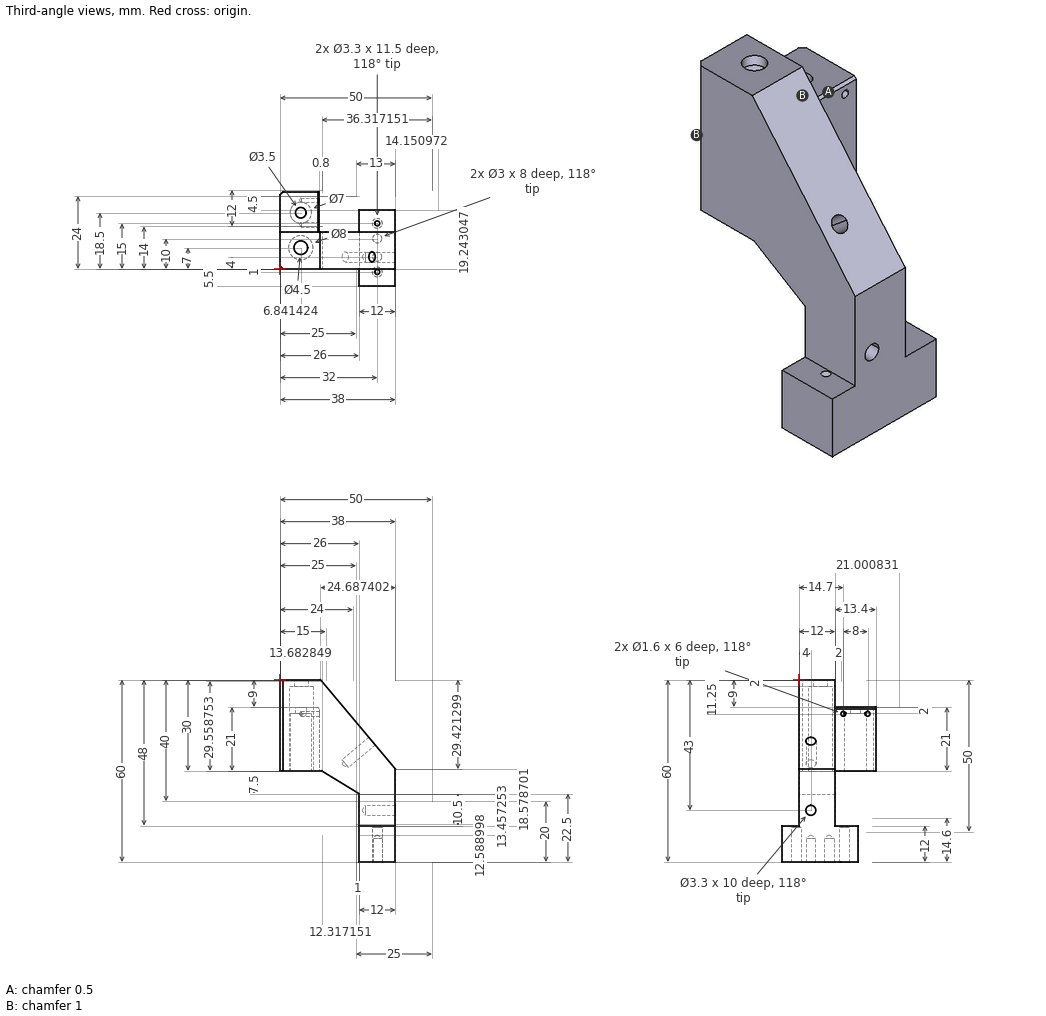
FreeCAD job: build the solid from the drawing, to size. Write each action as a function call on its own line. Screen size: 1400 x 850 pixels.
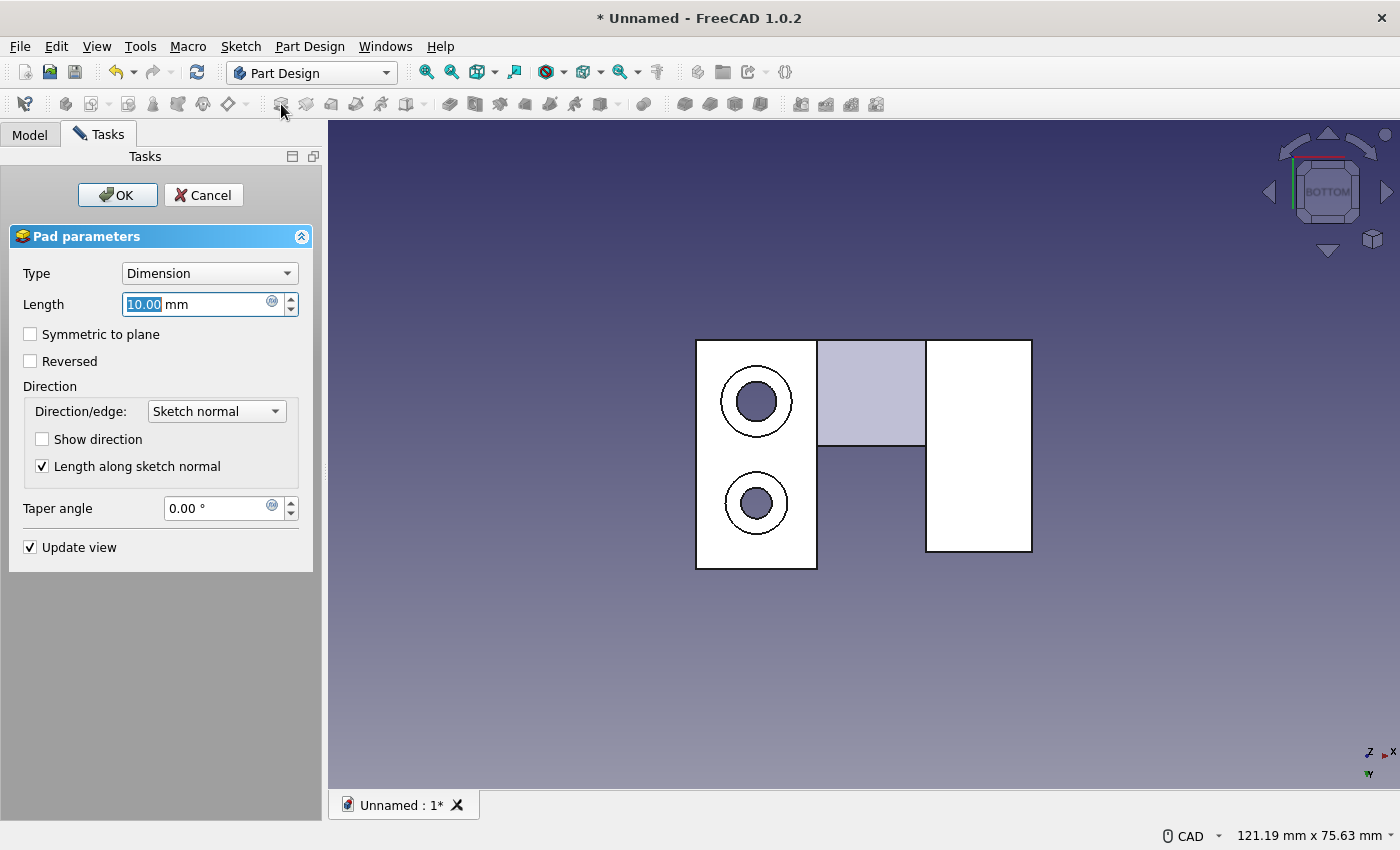
text(12)
key(Tab)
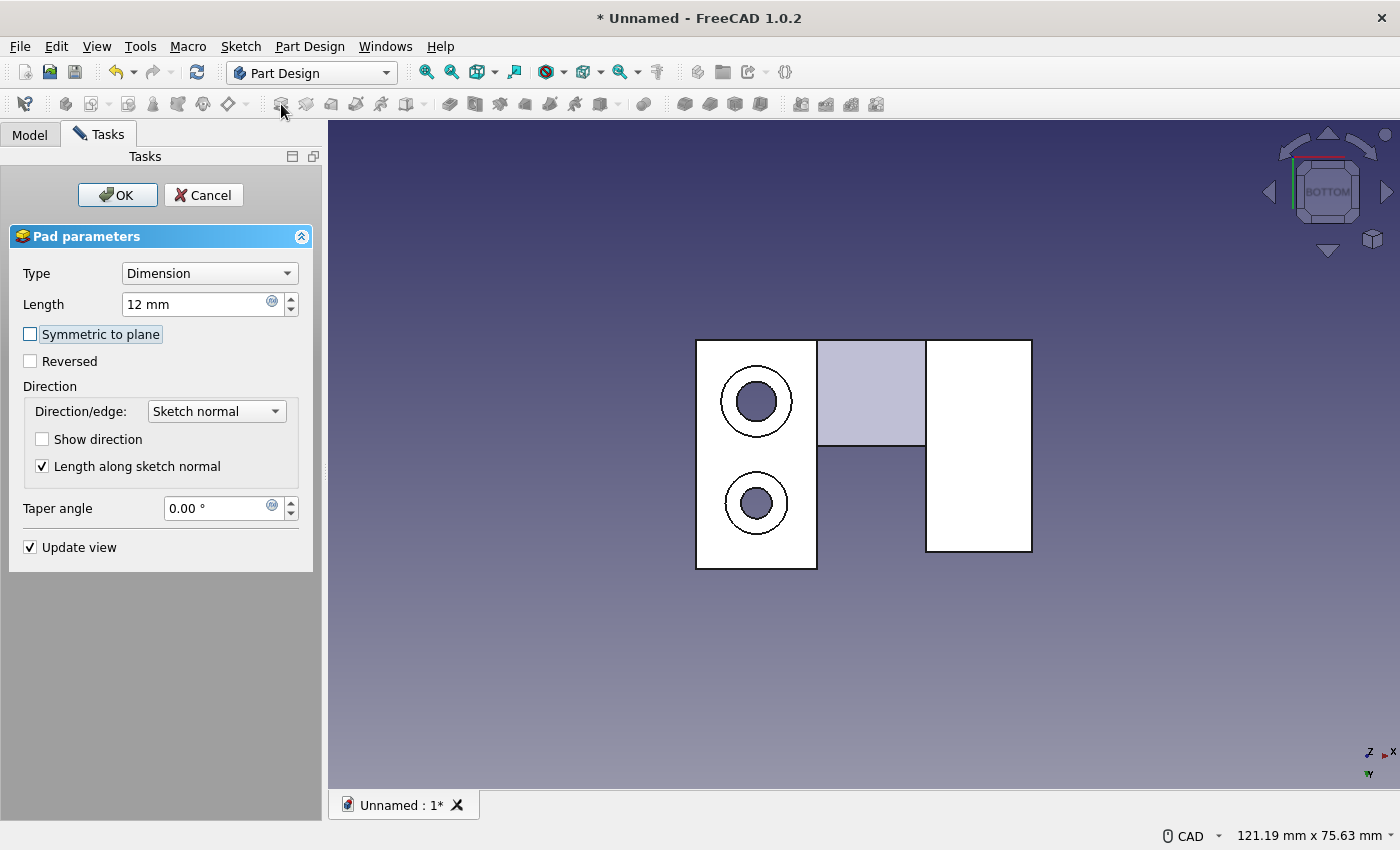
click(31, 361)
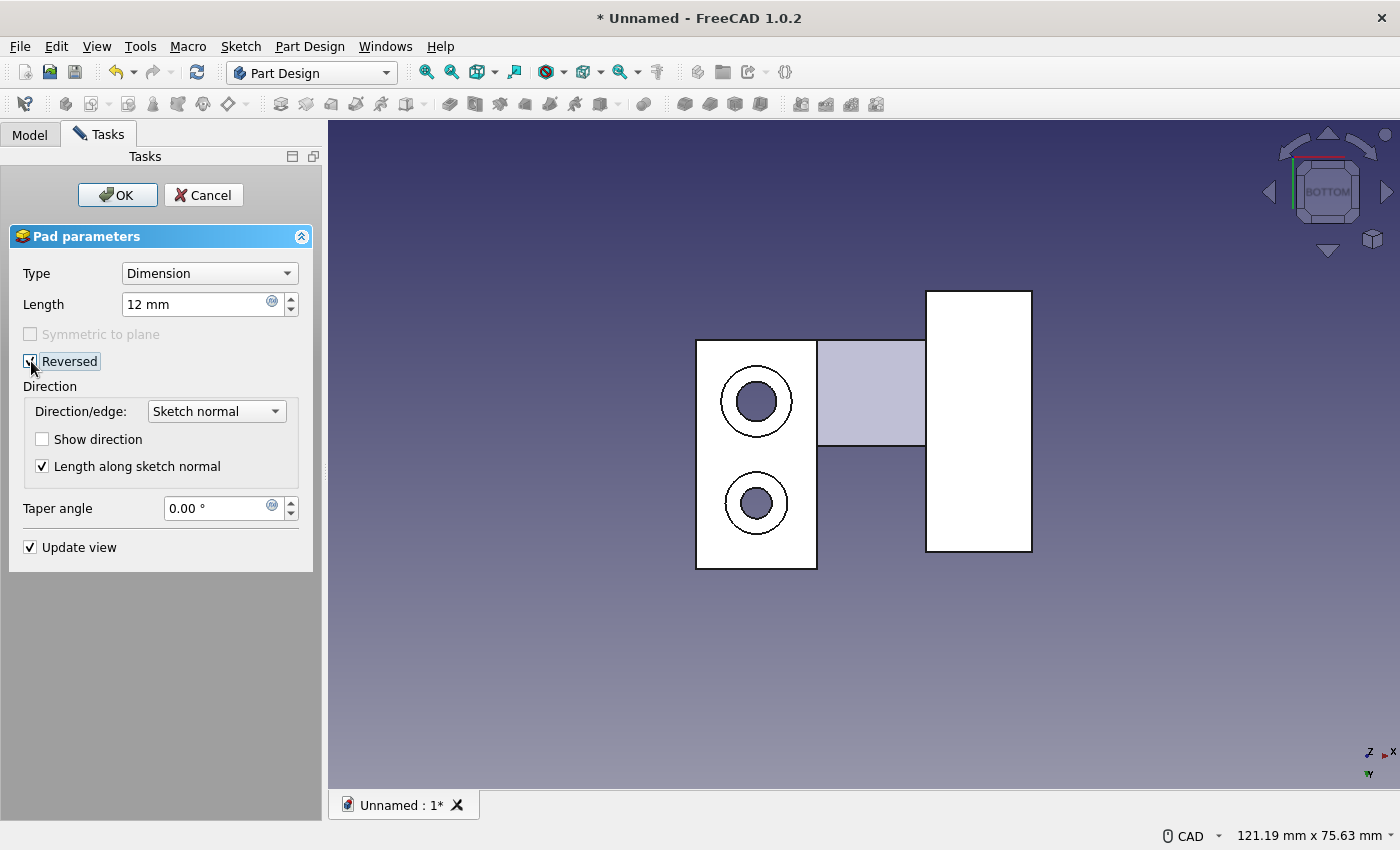
click(118, 195)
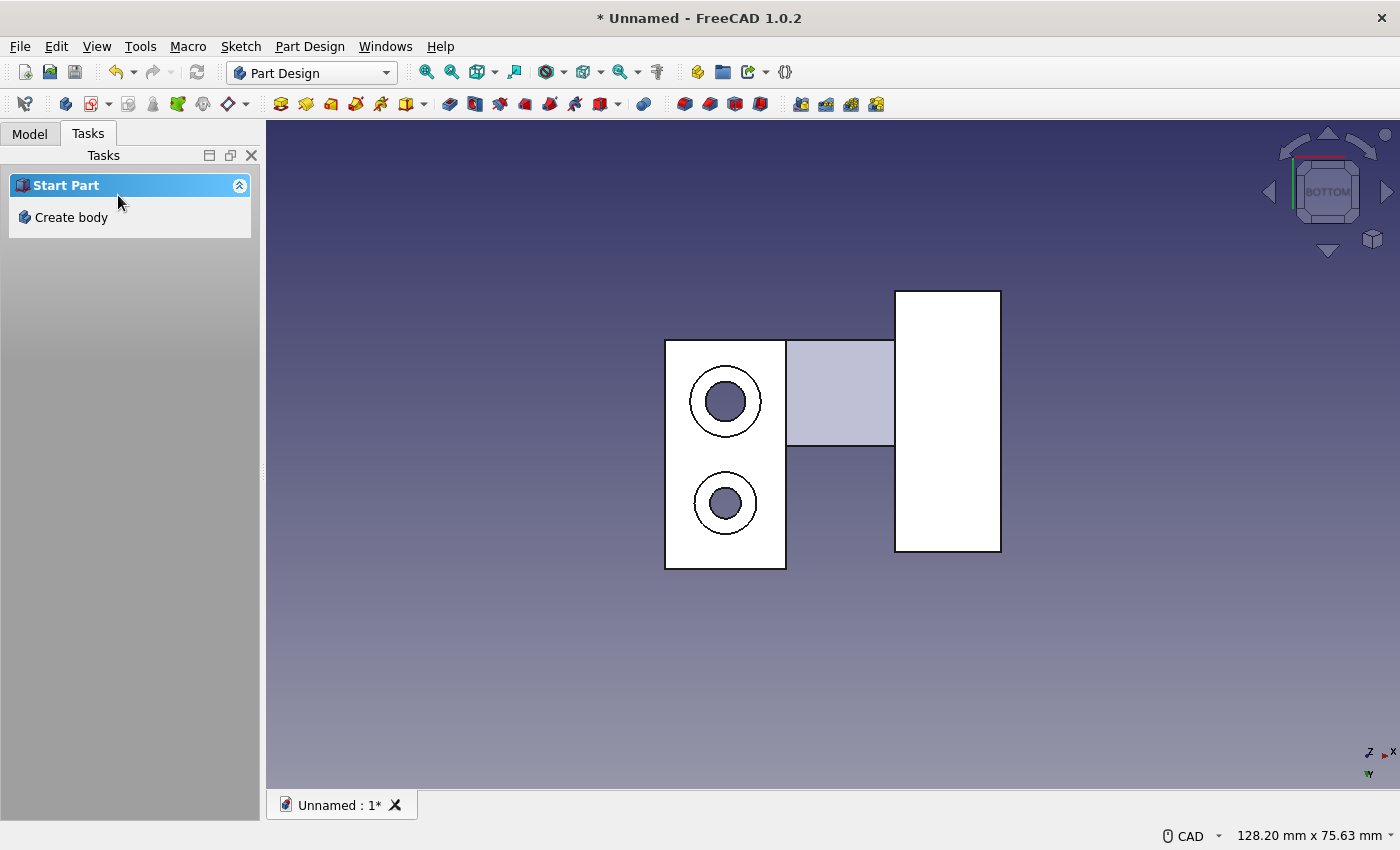
click(427, 72)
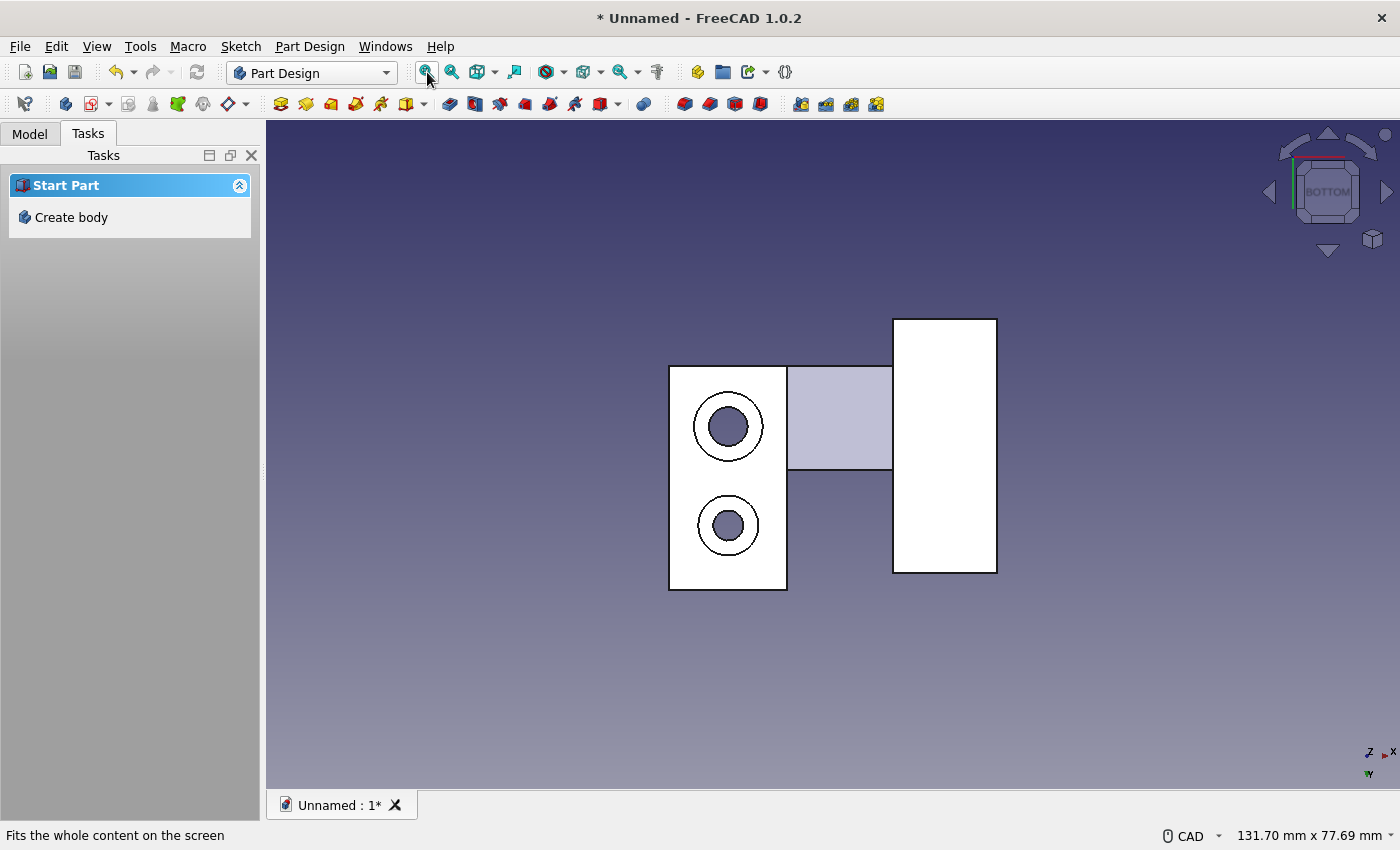
click(945, 517)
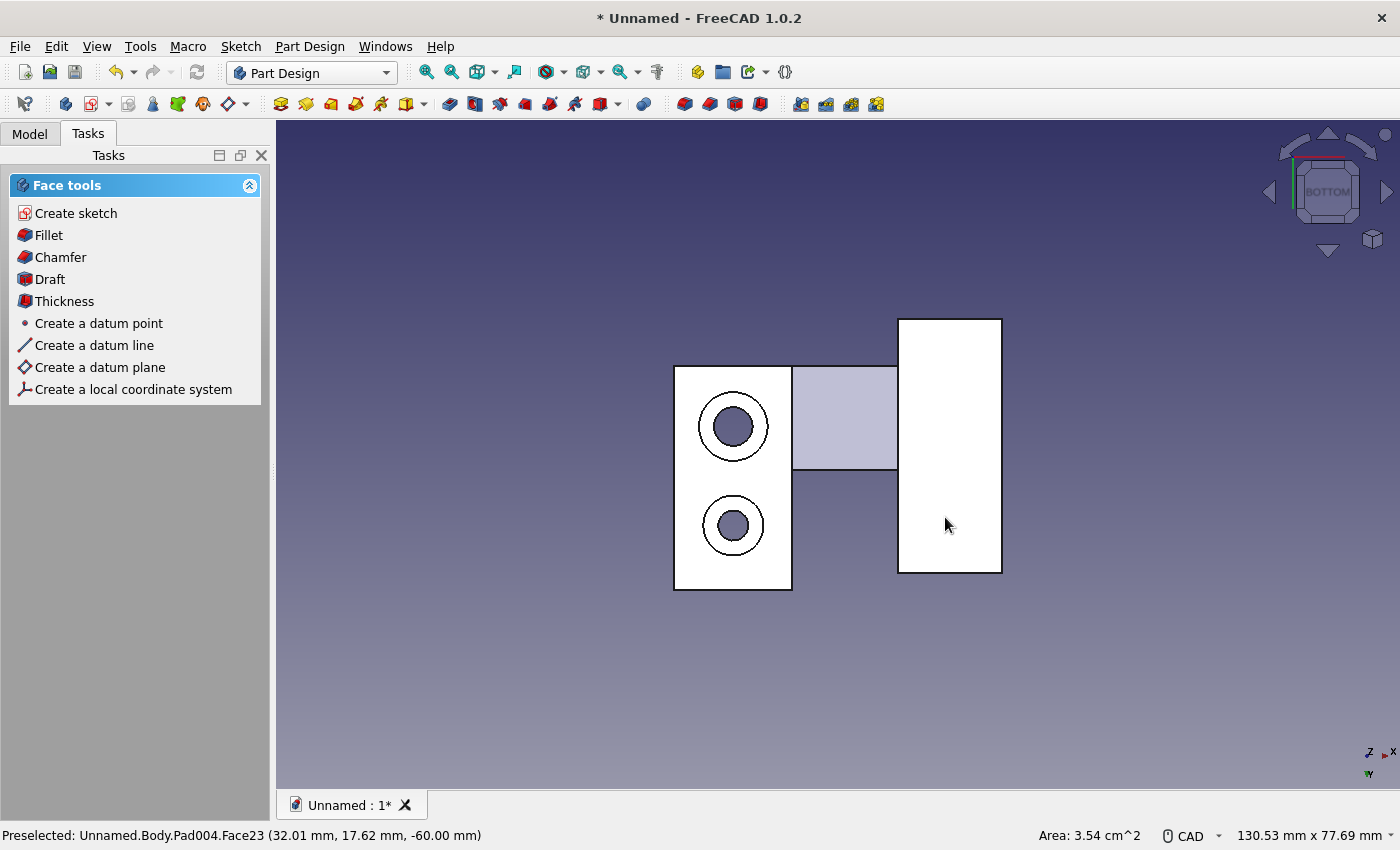
click(90, 104)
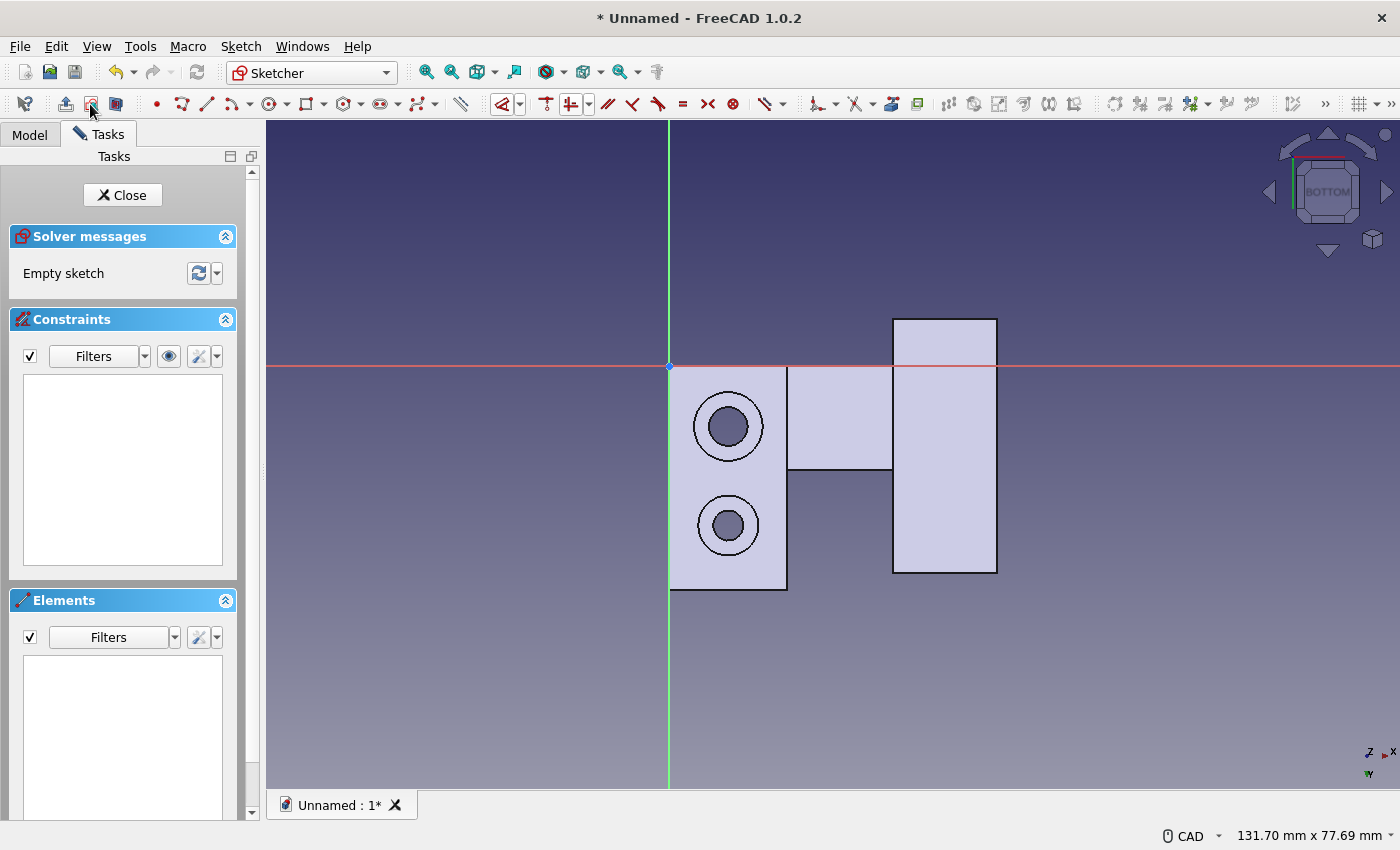
scroll(981, 573, up, 9)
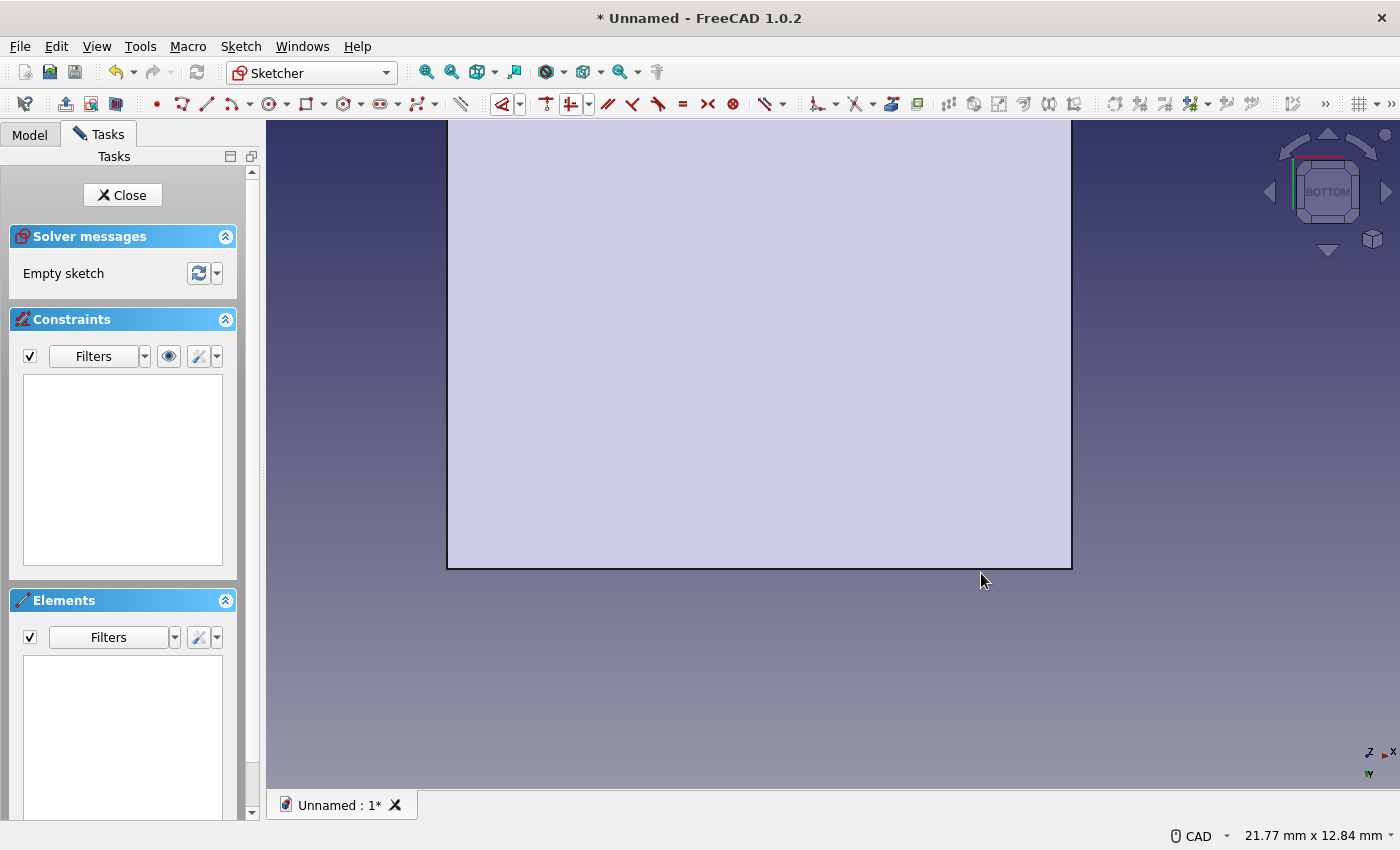
click(306, 104)